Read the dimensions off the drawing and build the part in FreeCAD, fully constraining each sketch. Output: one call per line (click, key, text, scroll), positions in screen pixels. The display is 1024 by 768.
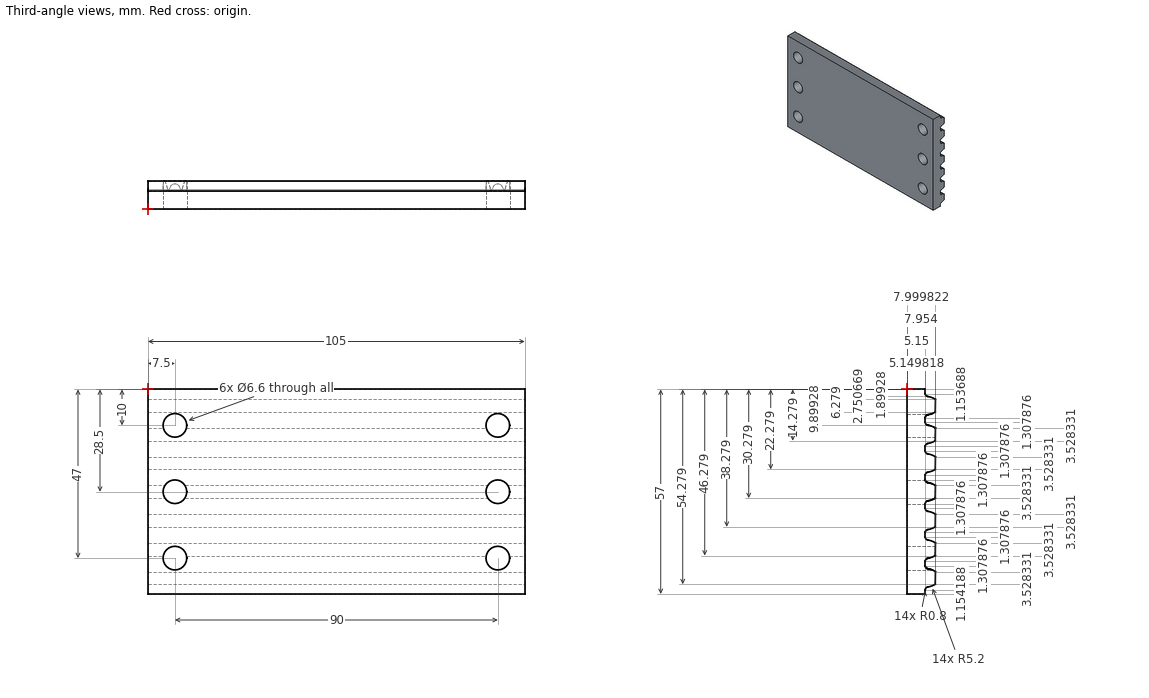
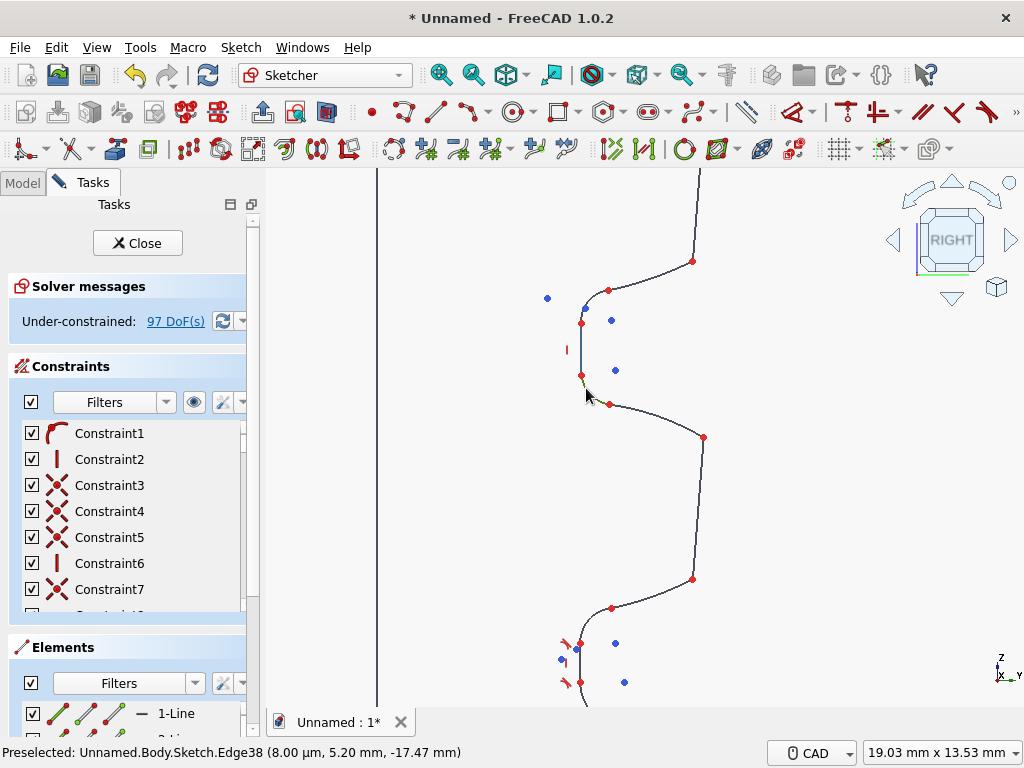
click(988, 112)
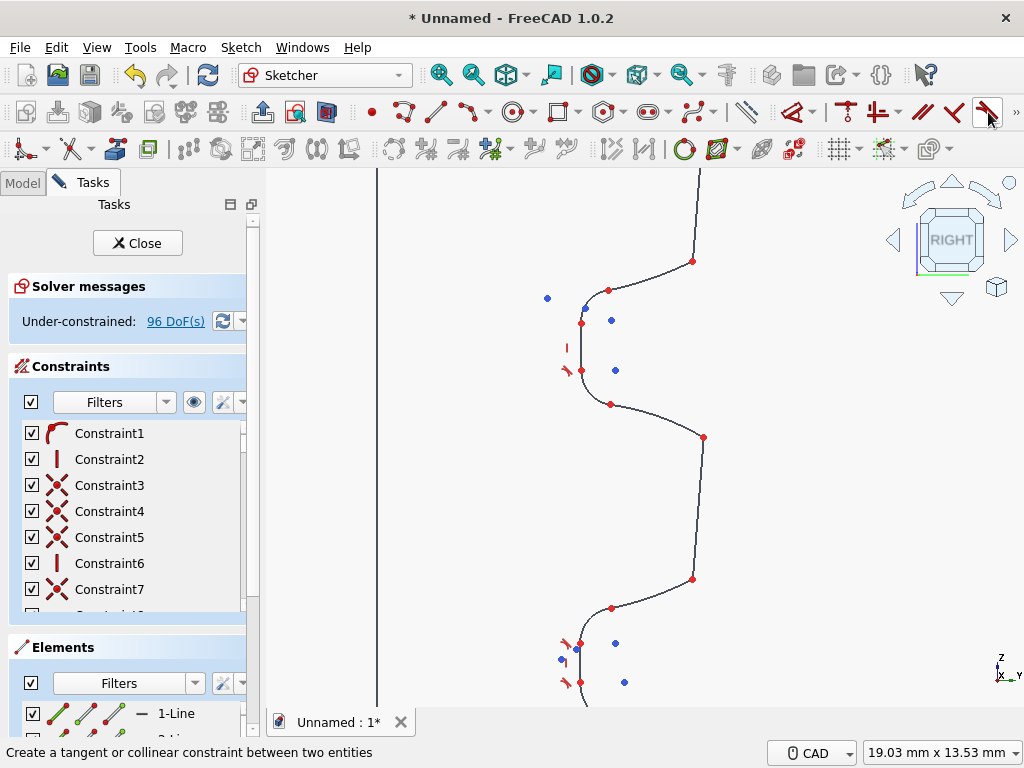
click(581, 357)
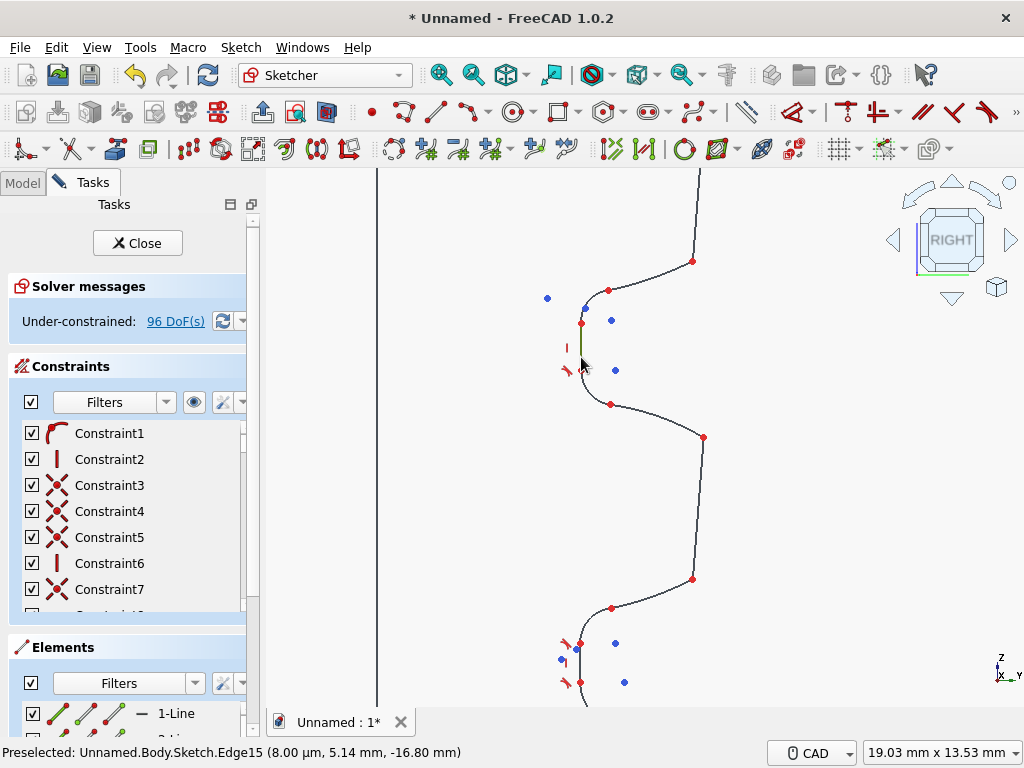
click(595, 295)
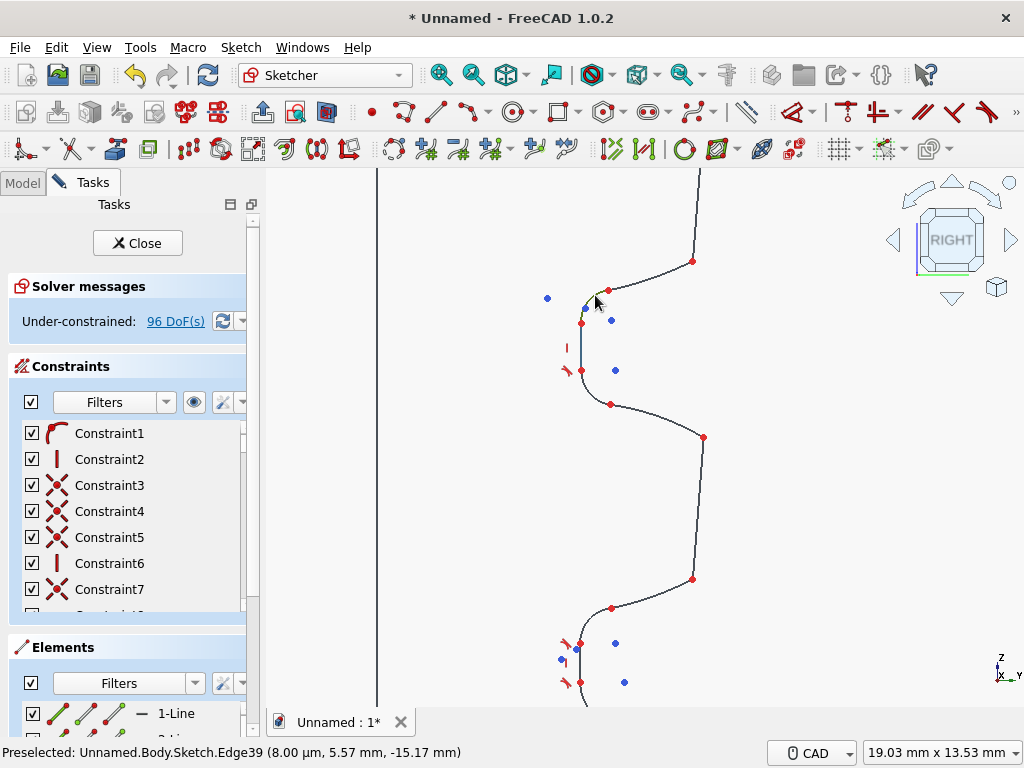
click(988, 112)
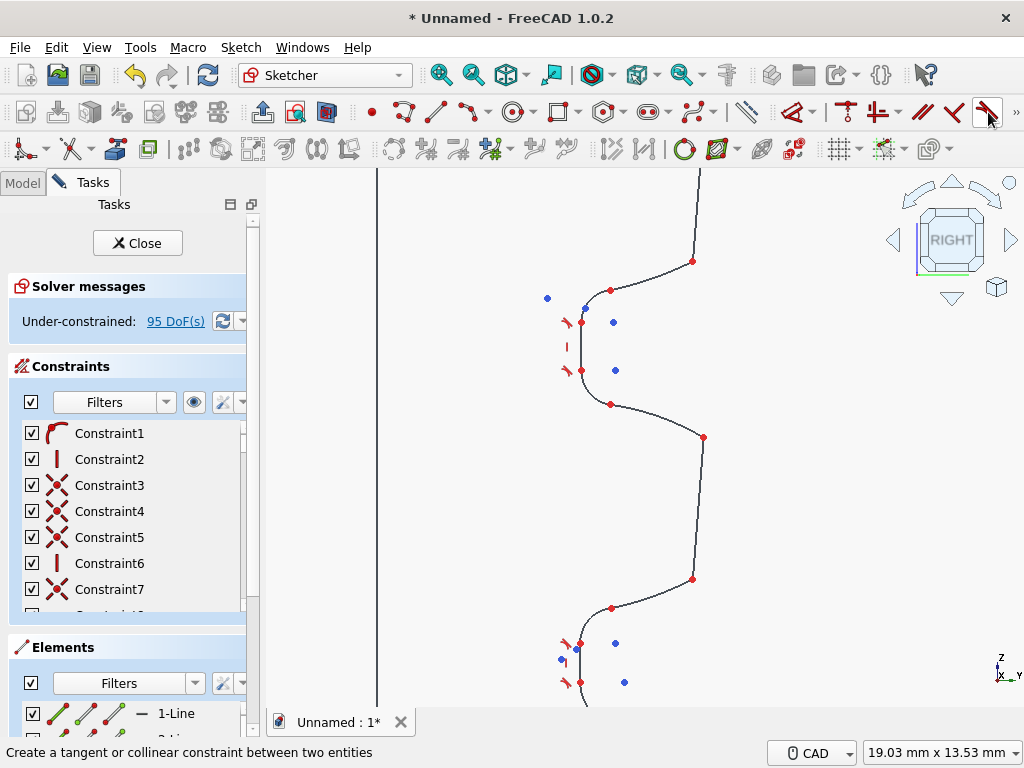
scroll(585, 361, down, 9)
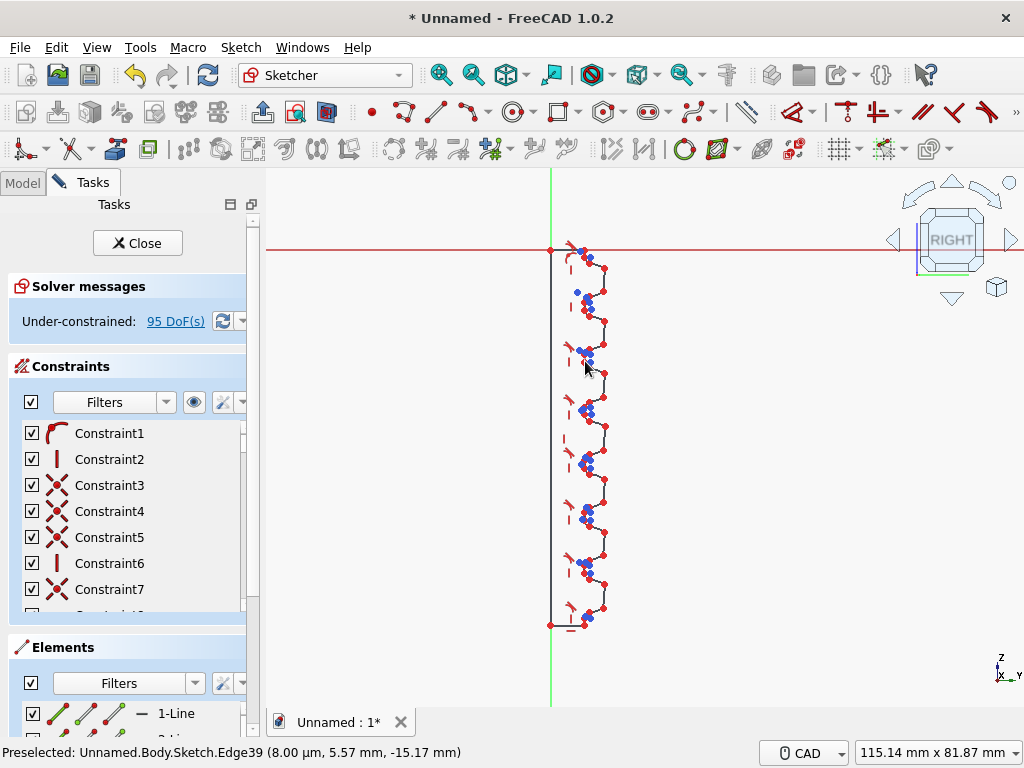
scroll(585, 308, up, 9)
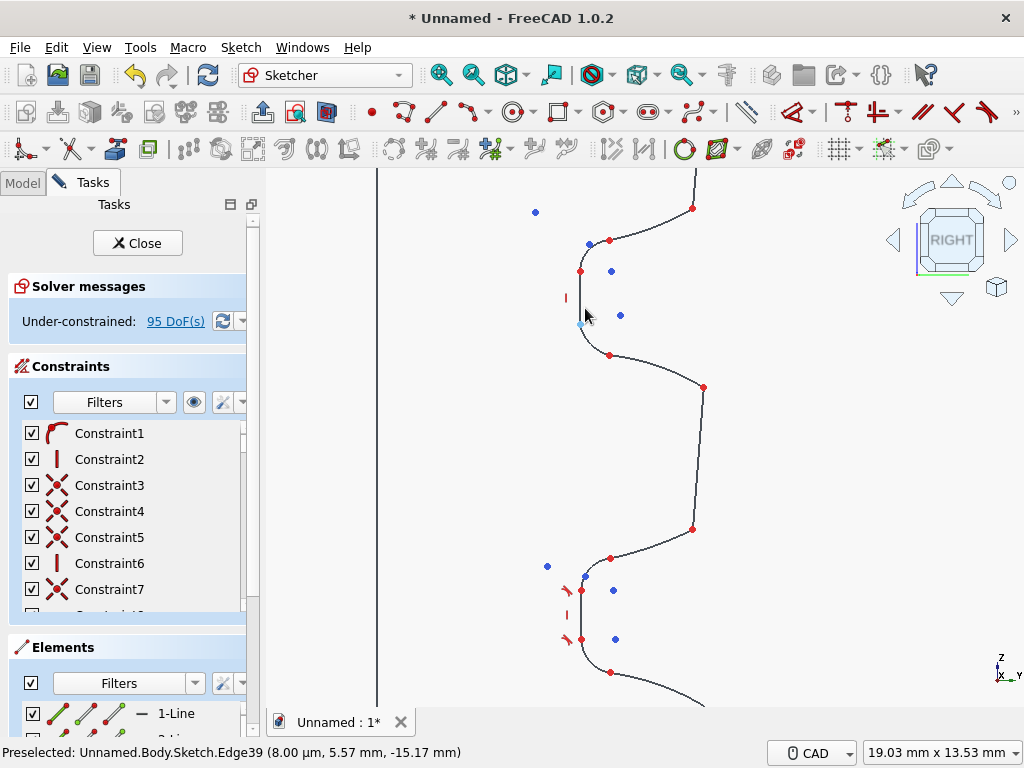
click(580, 309)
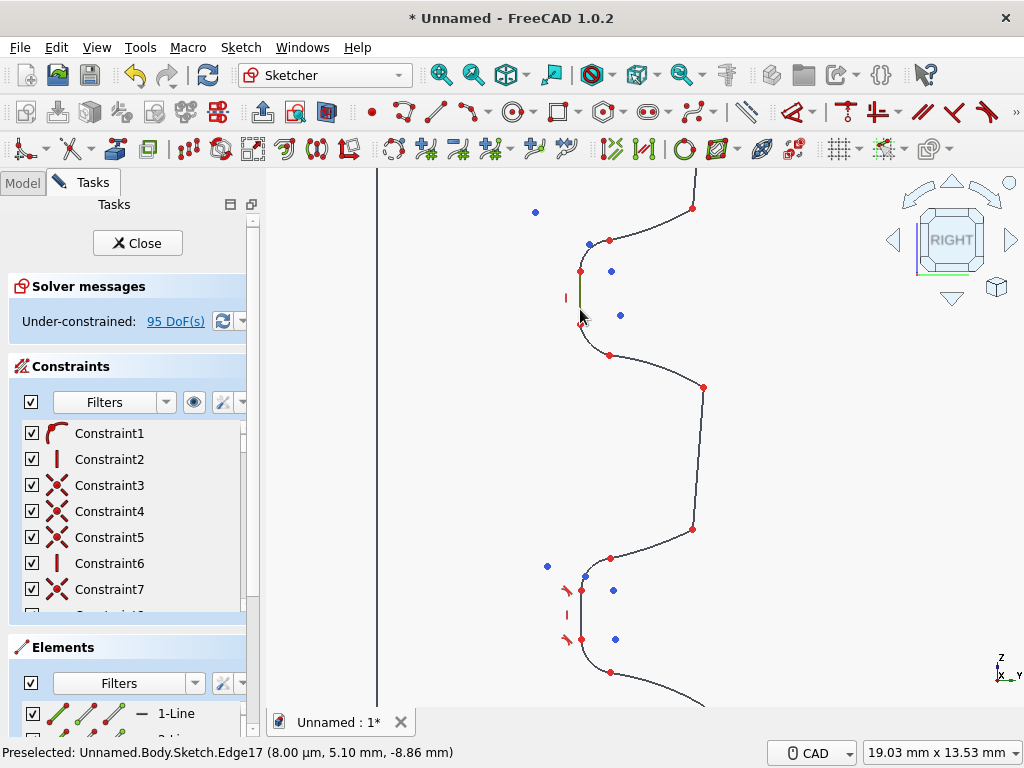
click(585, 337)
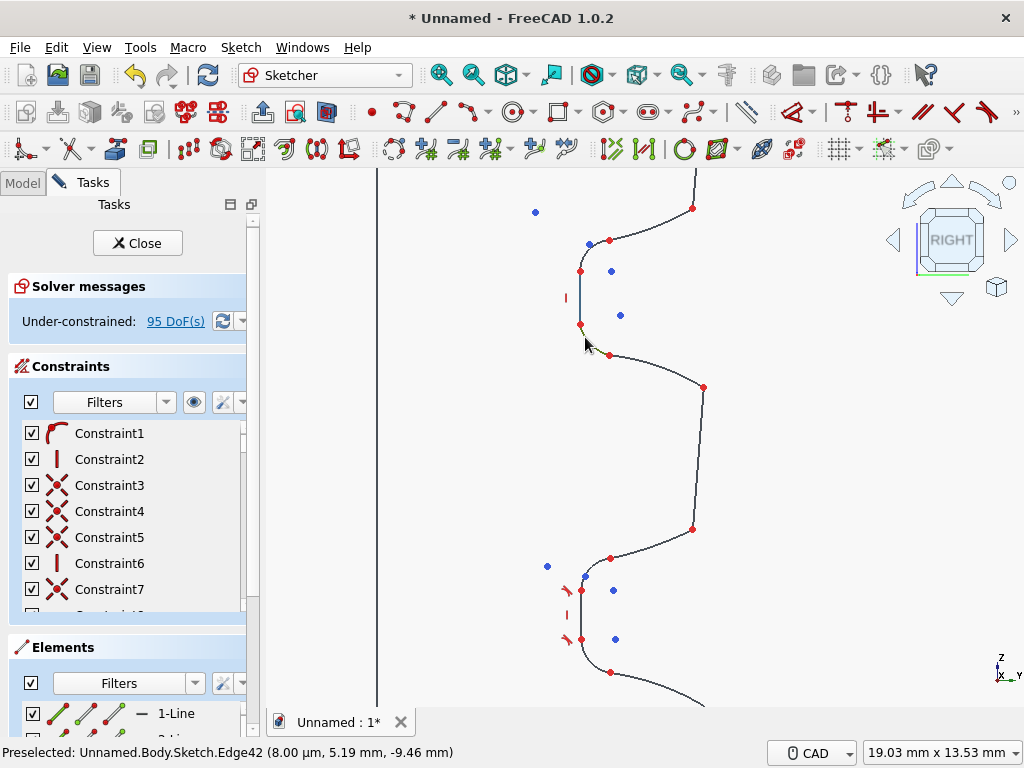
click(988, 112)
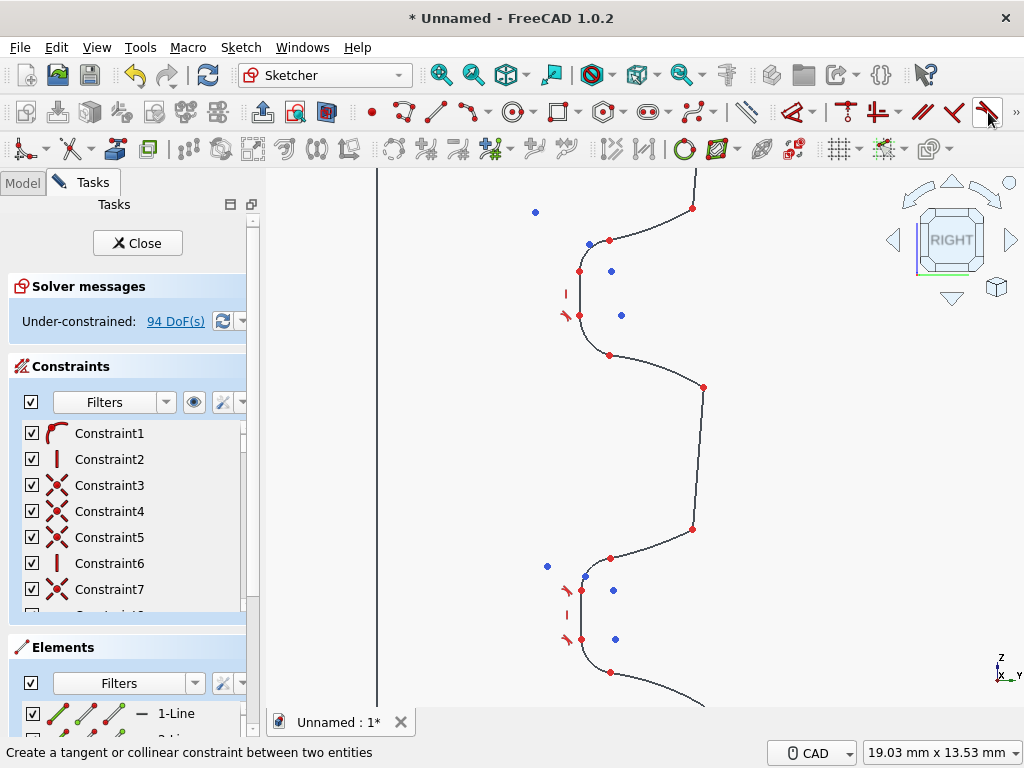
click(580, 302)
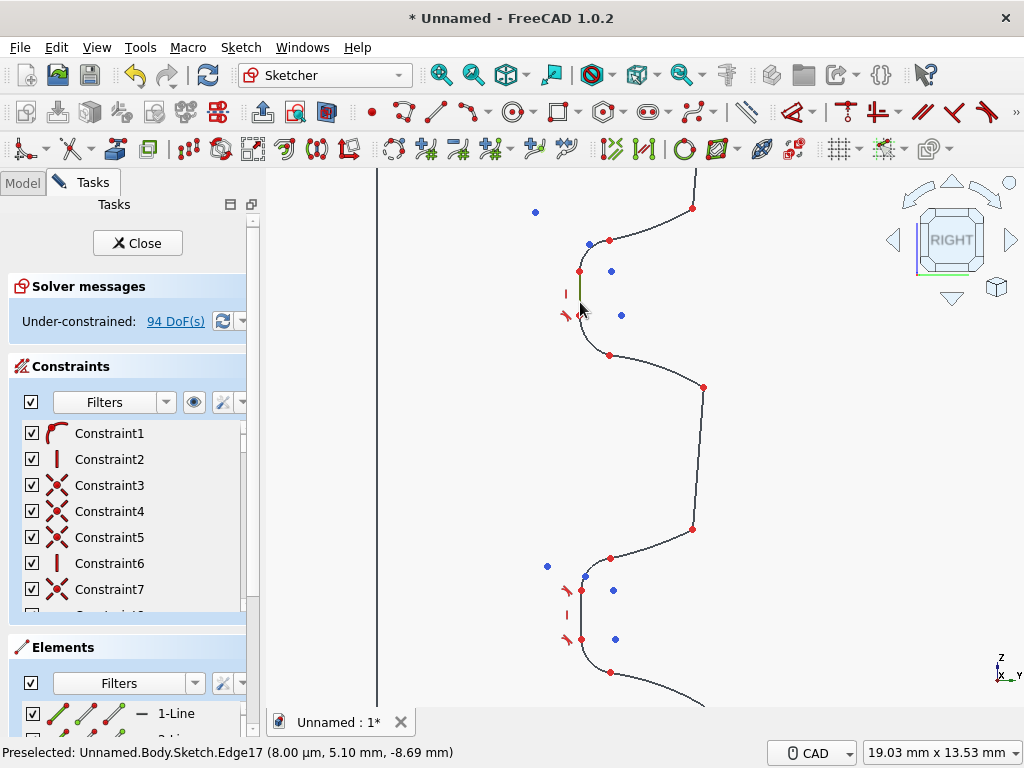
click(596, 244)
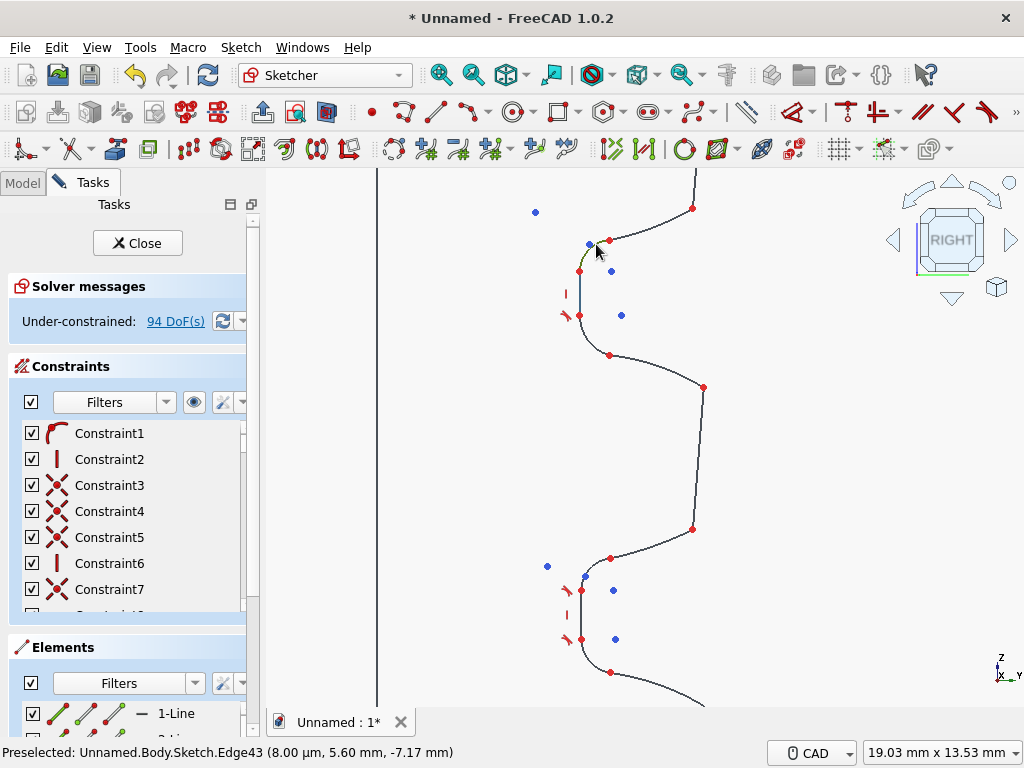
click(988, 112)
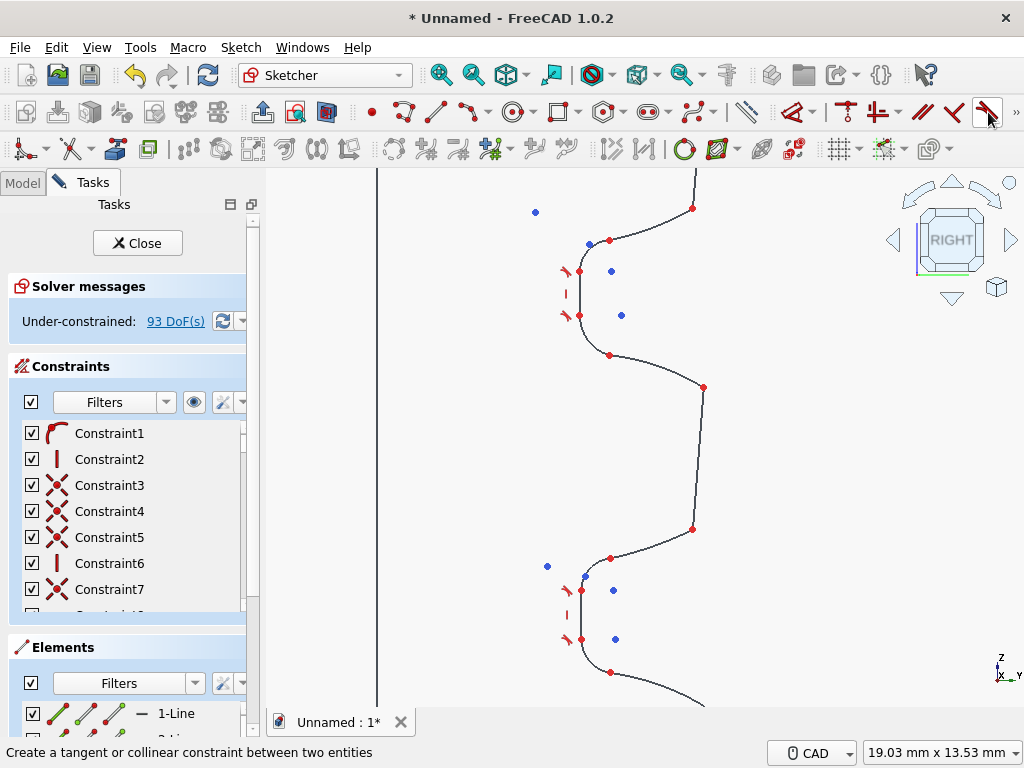
scroll(585, 308, down, 9)